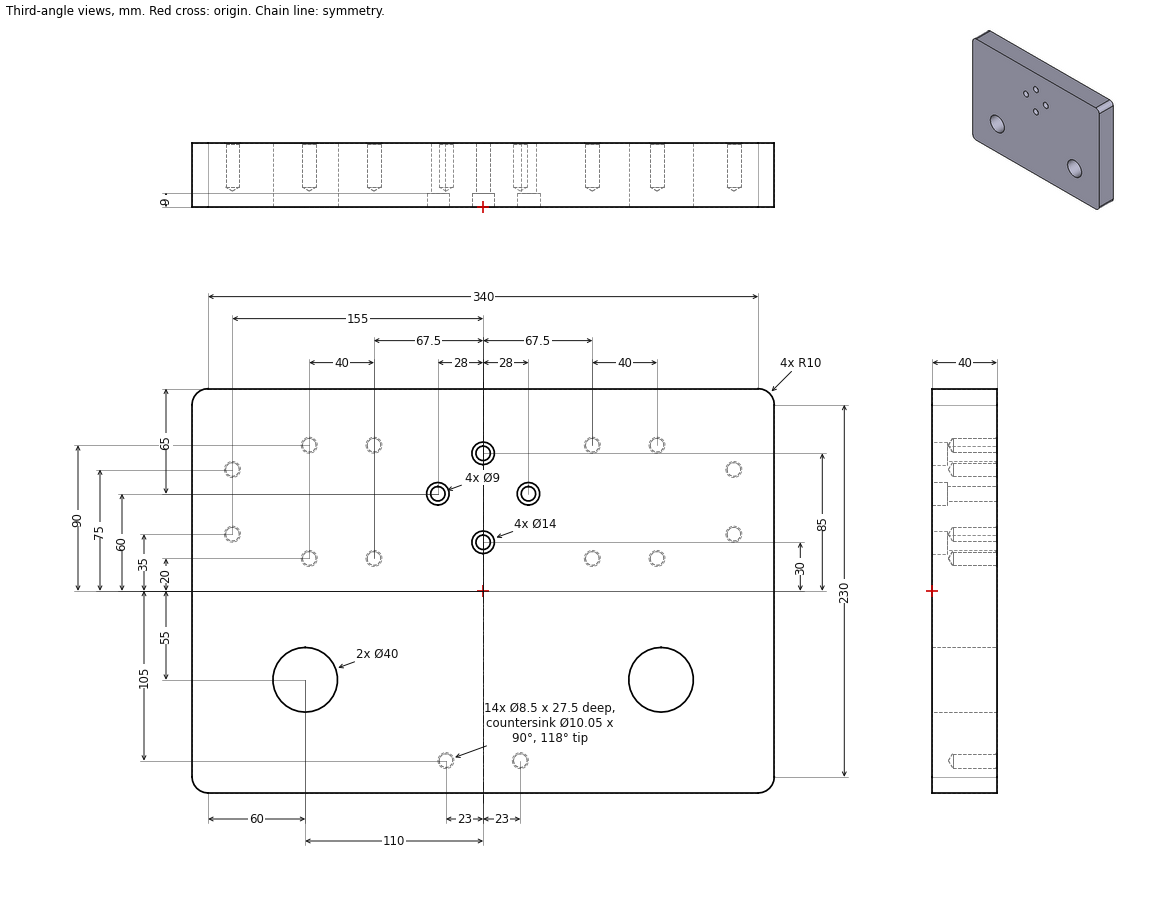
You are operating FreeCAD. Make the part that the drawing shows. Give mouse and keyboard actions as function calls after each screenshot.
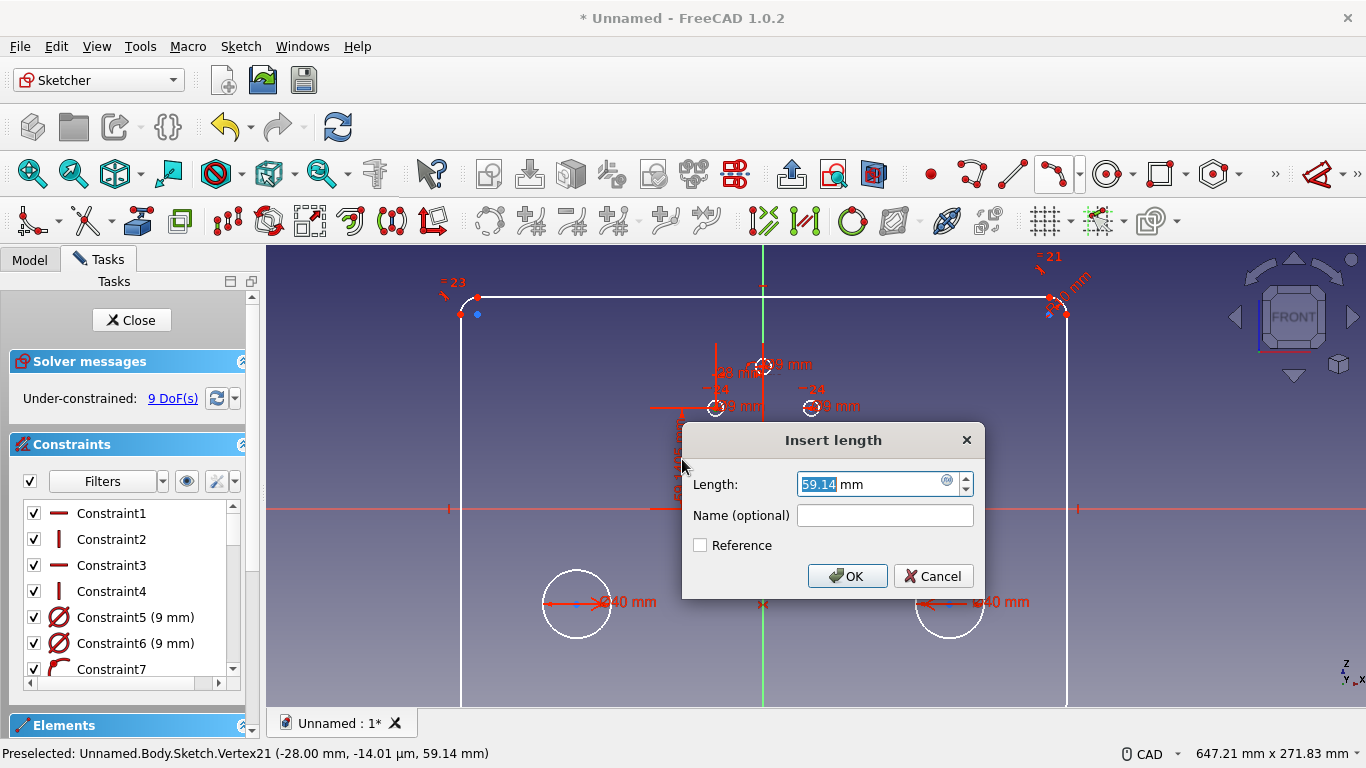
text(60)
key(Return)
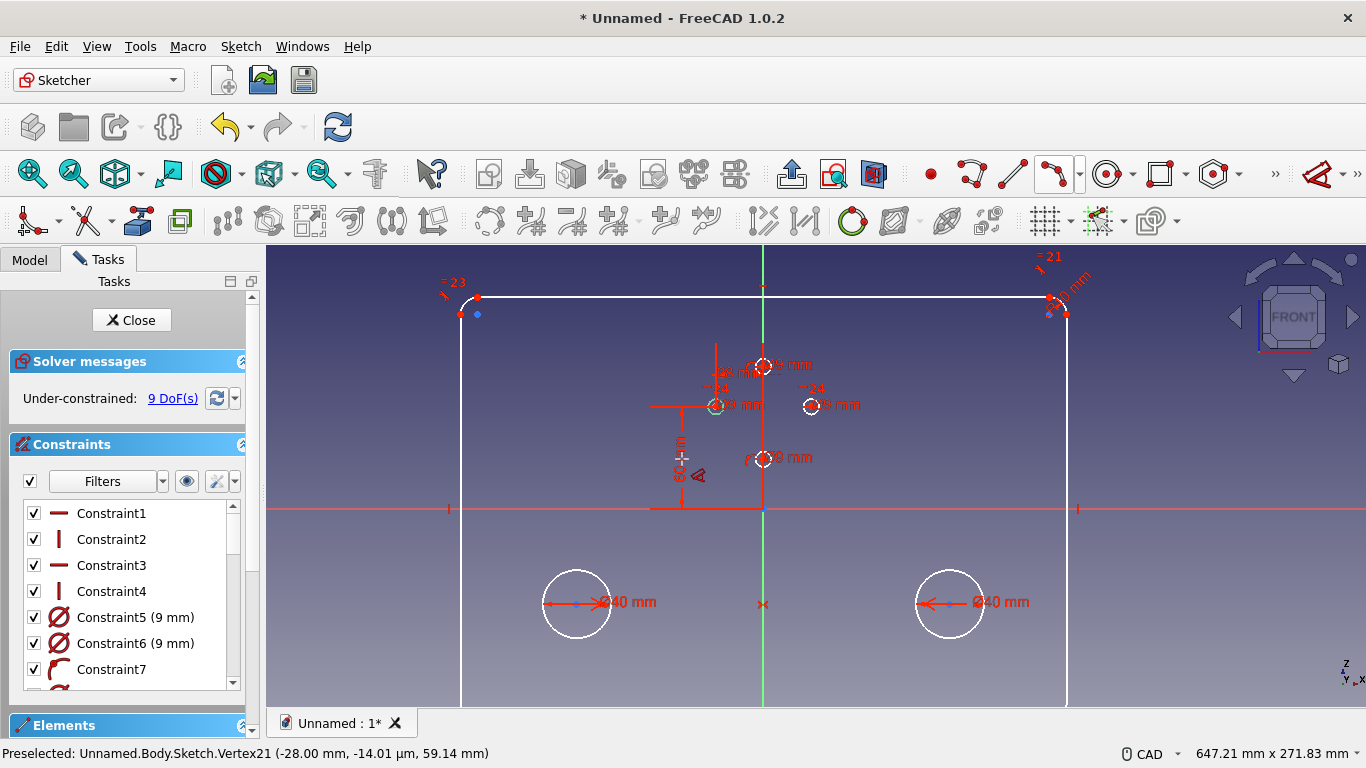
click(763, 367)
click(797, 438)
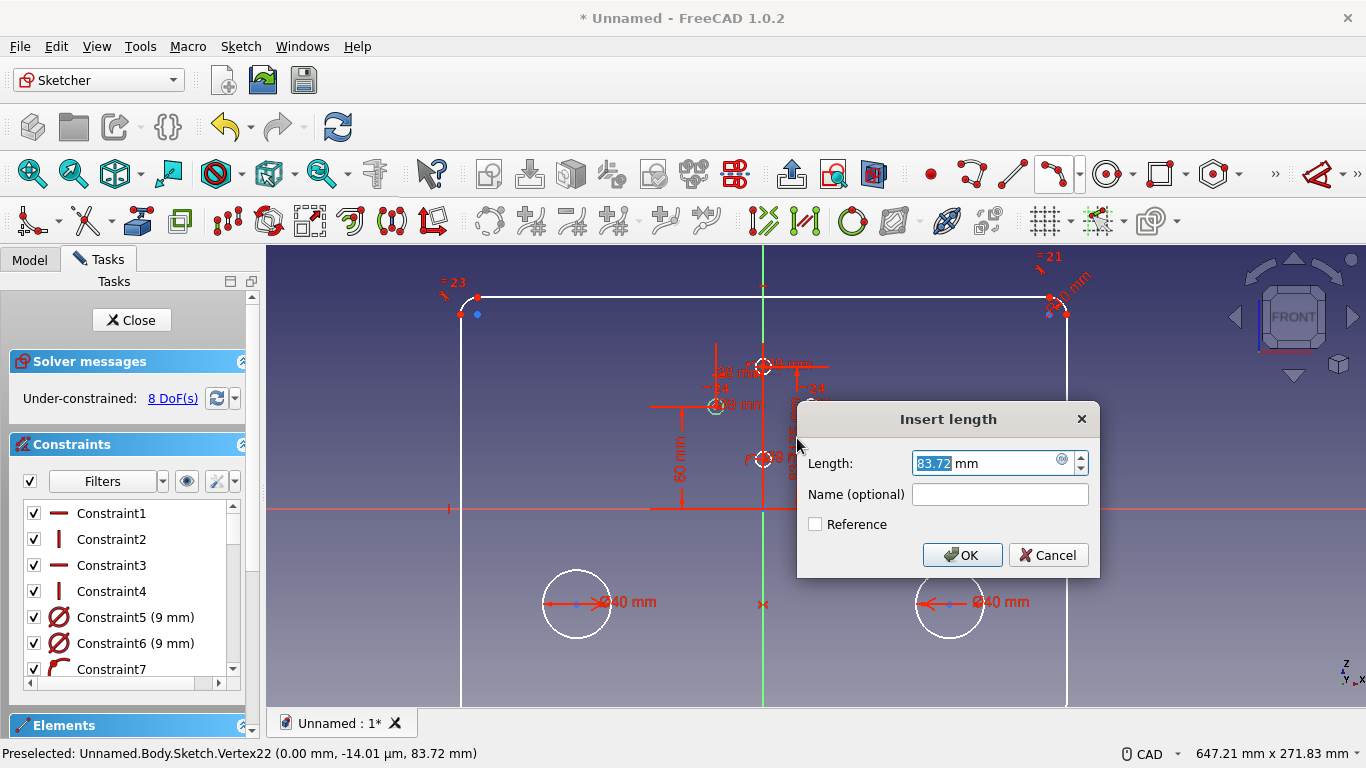
text(85)
key(Return)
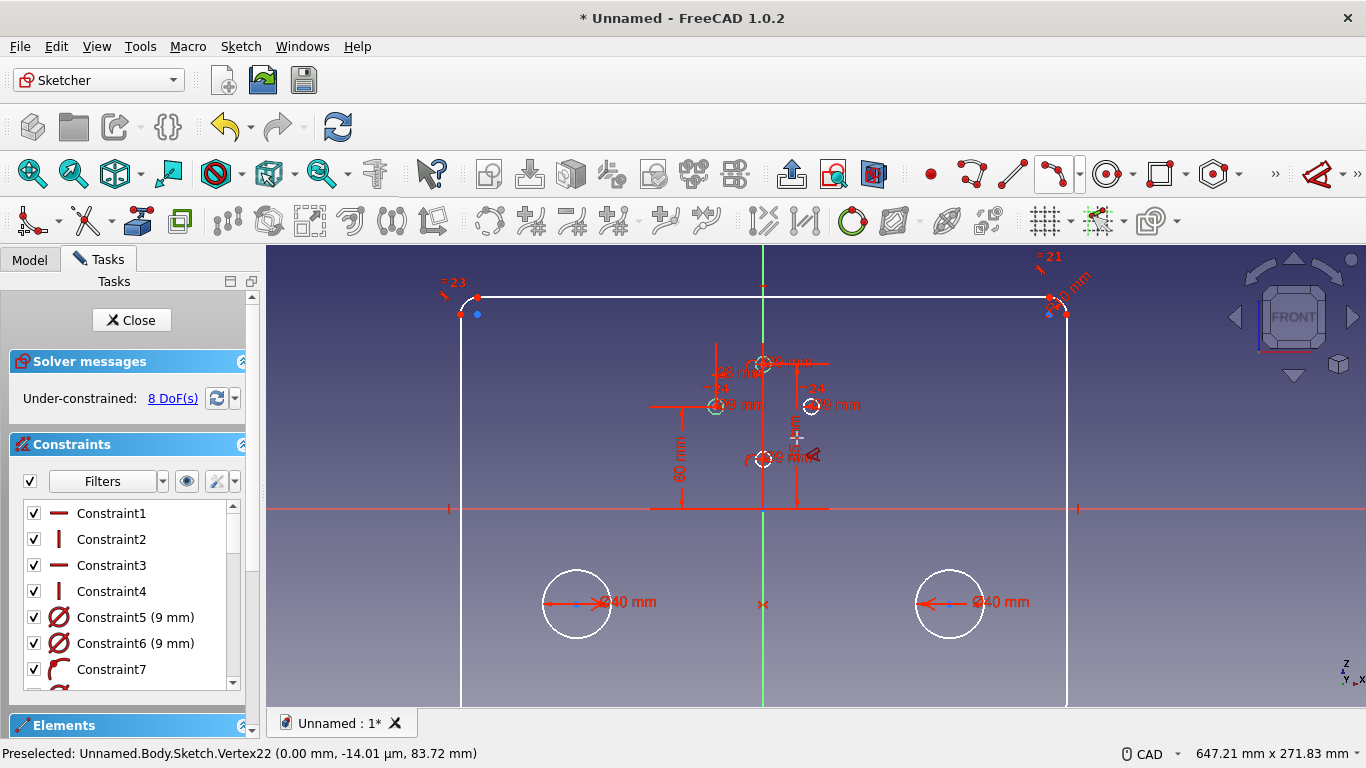
click(811, 407)
click(787, 543)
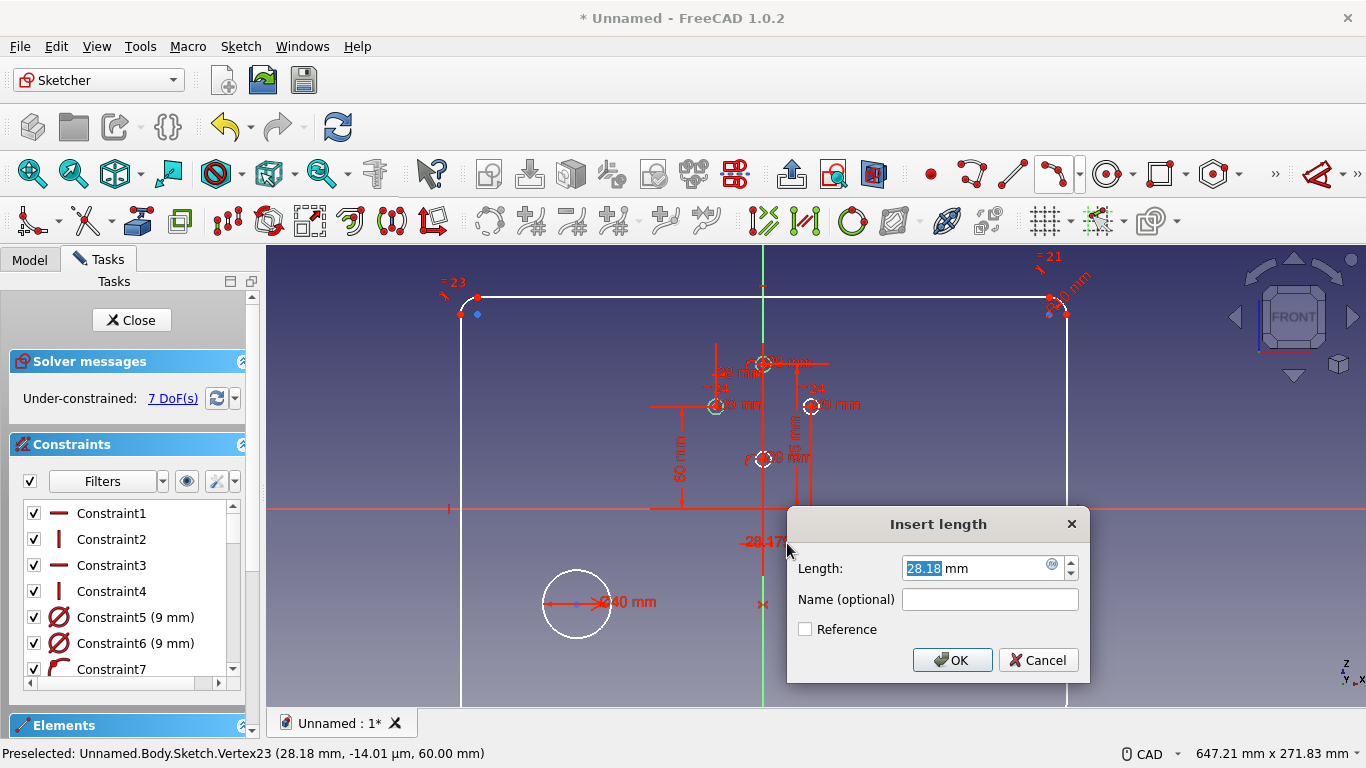
text(28)
key(Return)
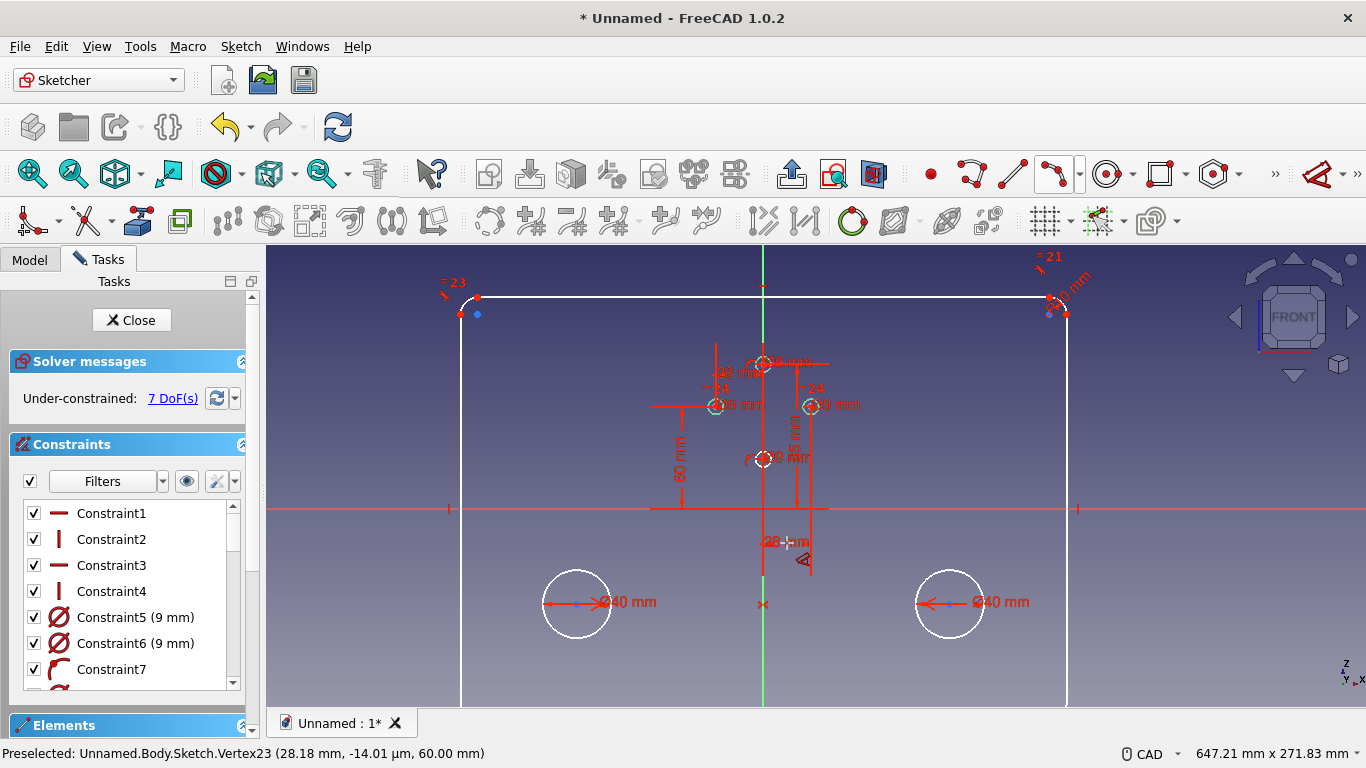
click(763, 459)
click(797, 484)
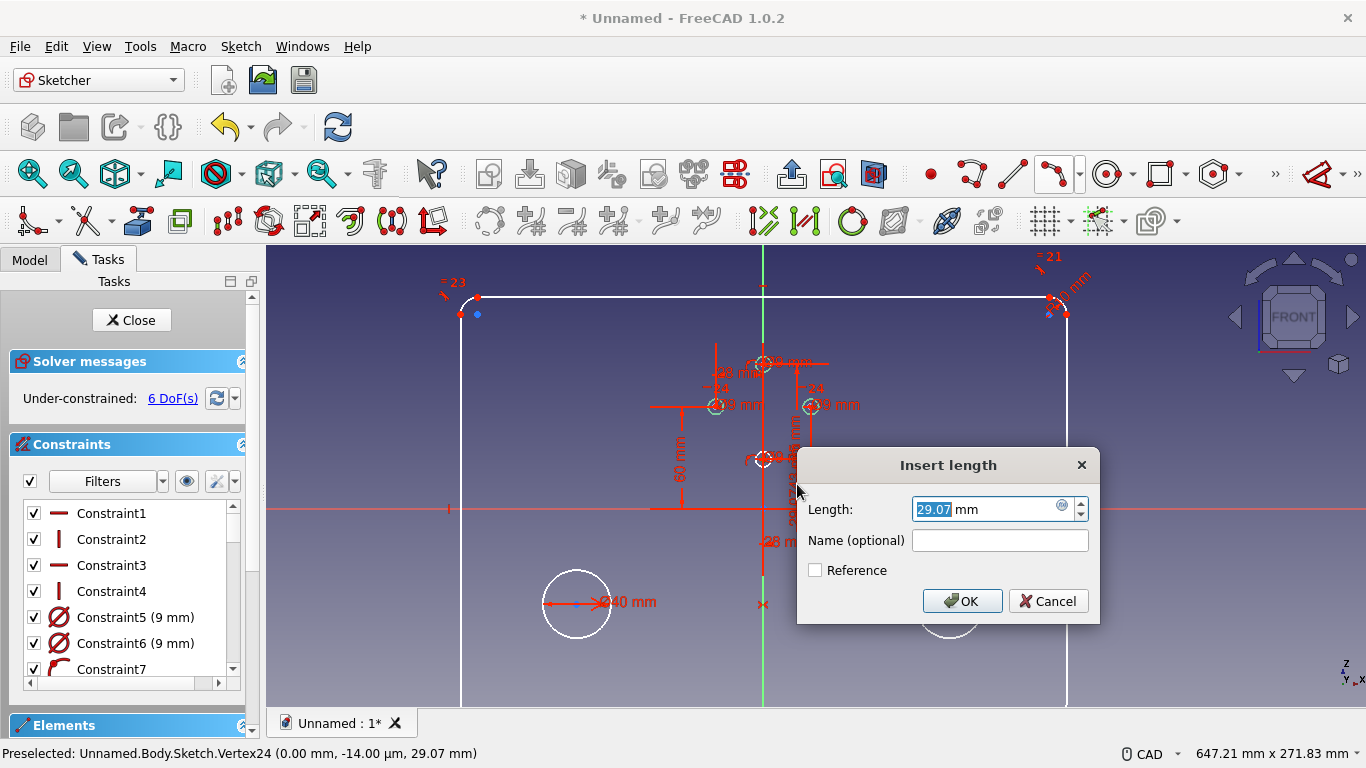
text(30)
key(Return)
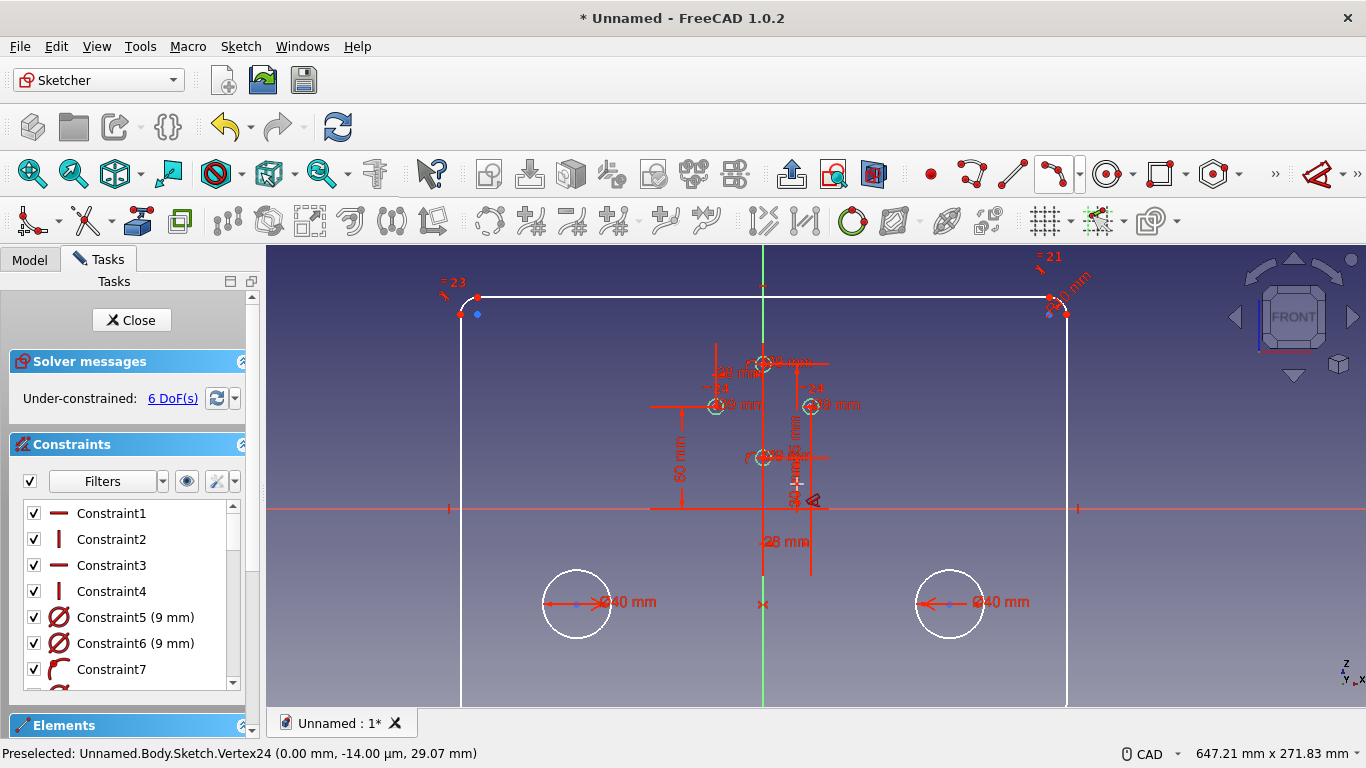
click(577, 604)
click(543, 556)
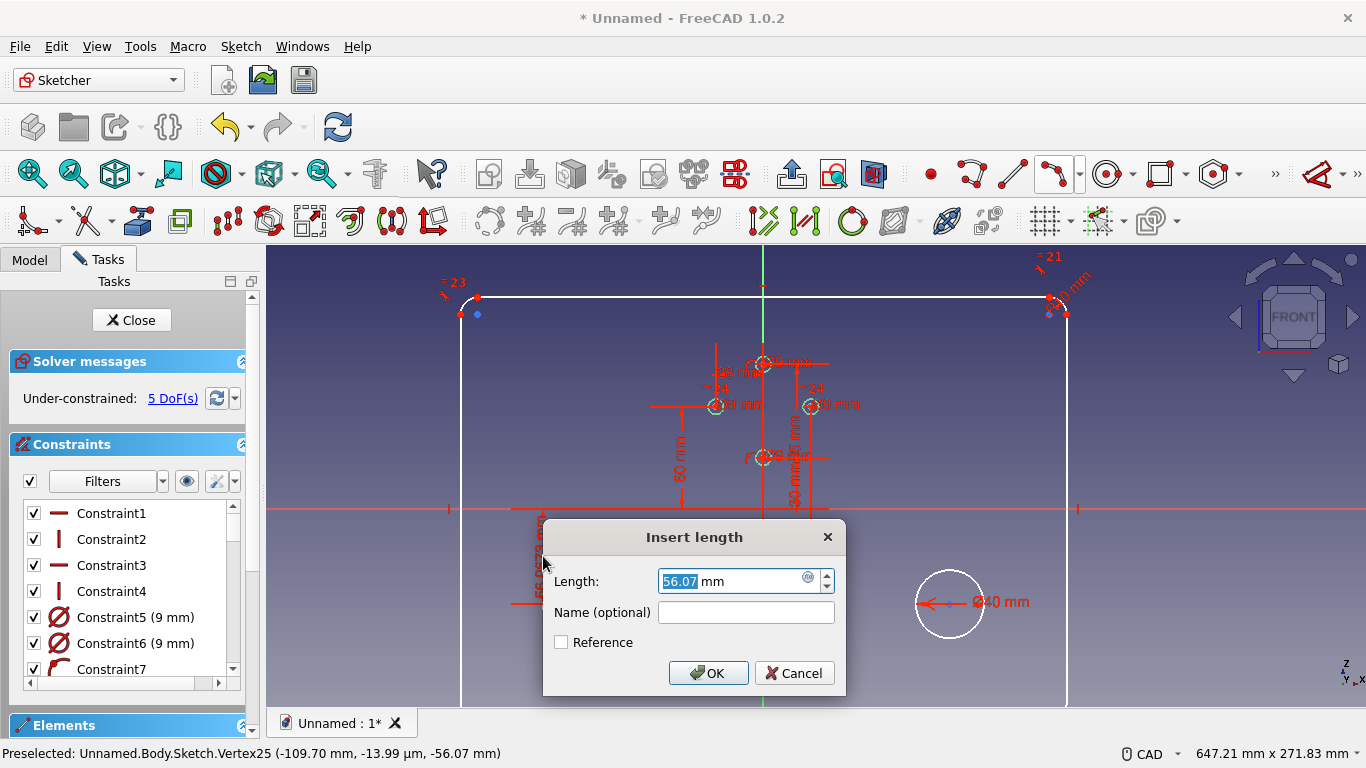
text(55)
key(Return)